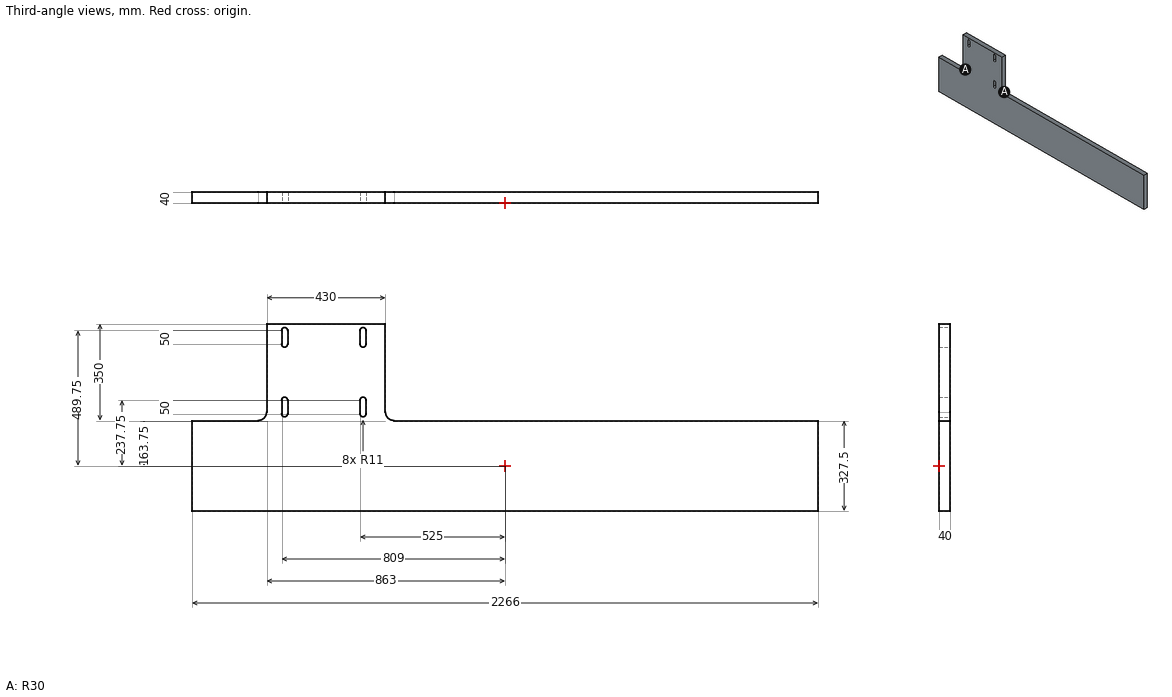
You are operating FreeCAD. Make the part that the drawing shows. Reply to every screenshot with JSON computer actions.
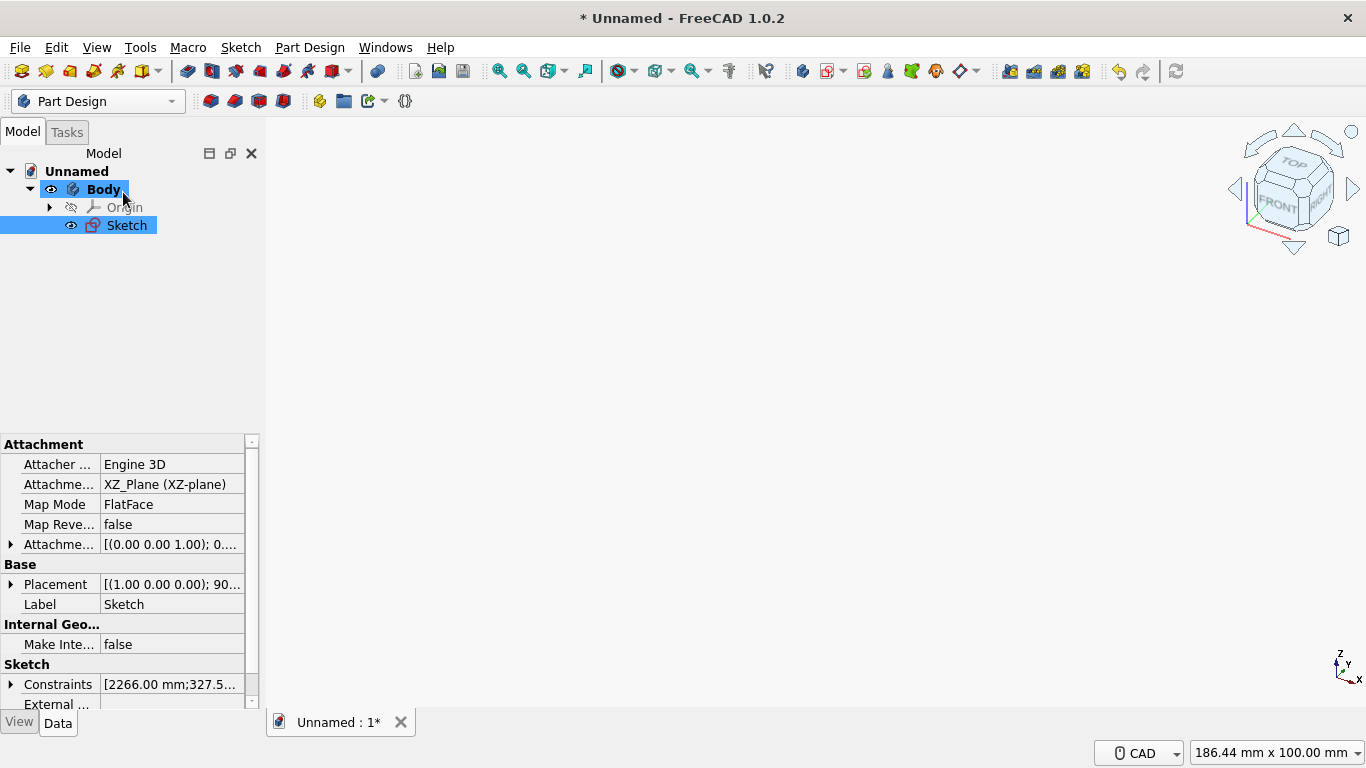
{"action": "left_click", "coordinate": [22, 72]}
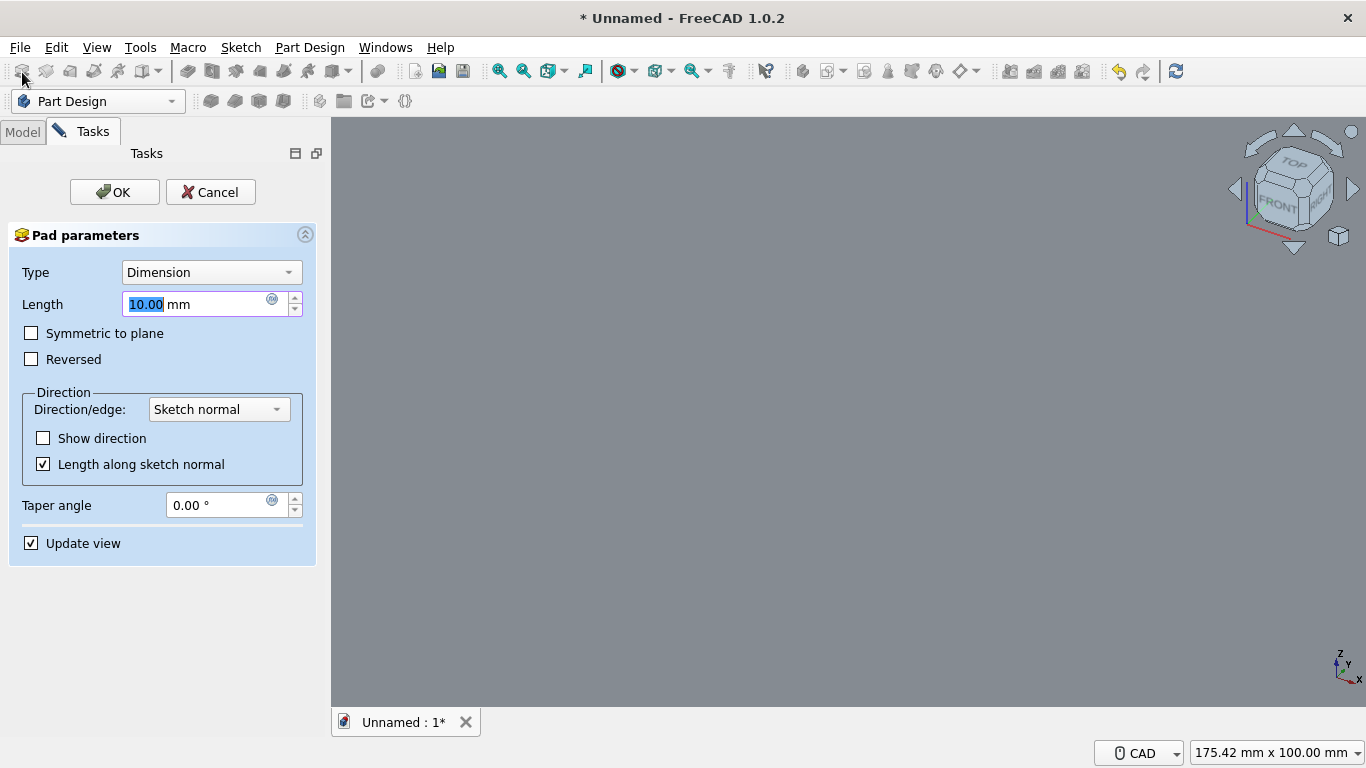
{"action": "type", "text": "40"}
{"action": "key", "text": "Tab"}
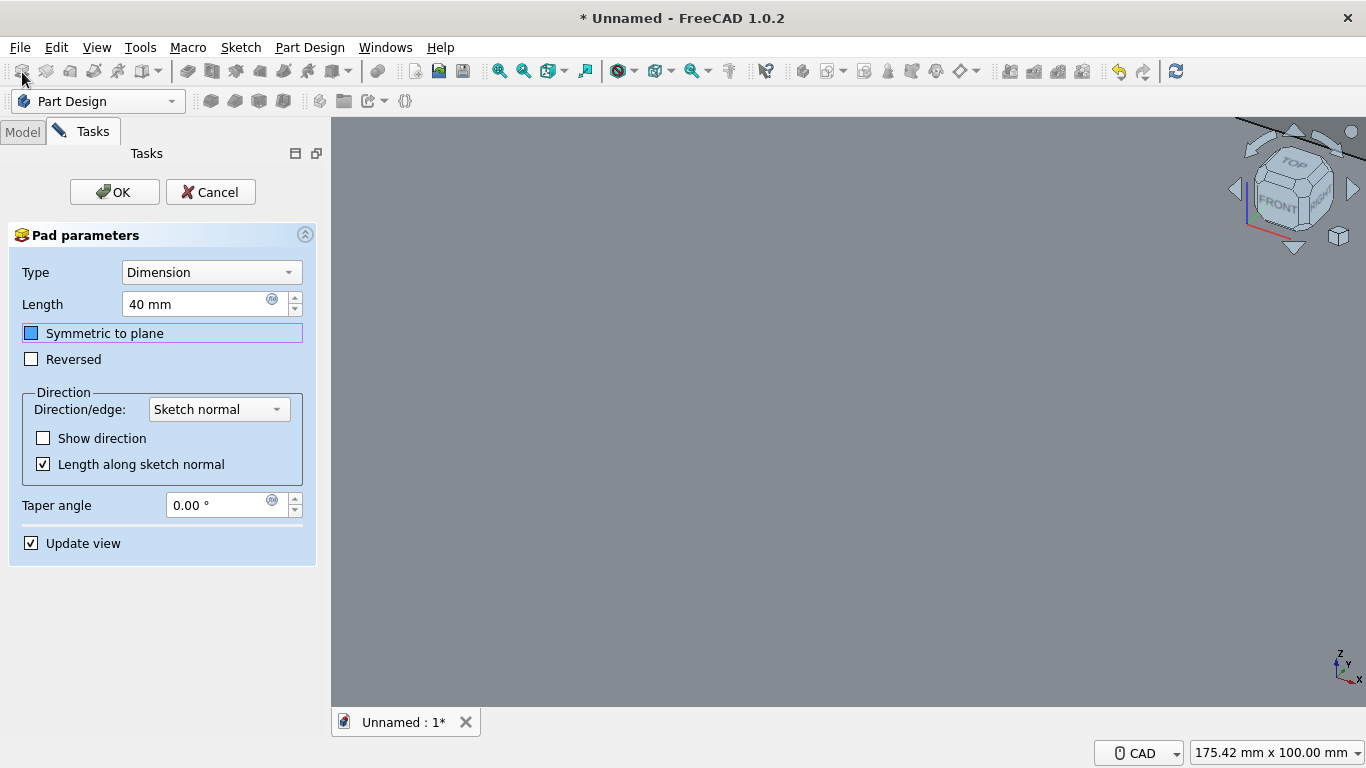
{"action": "left_click", "coordinate": [30, 359]}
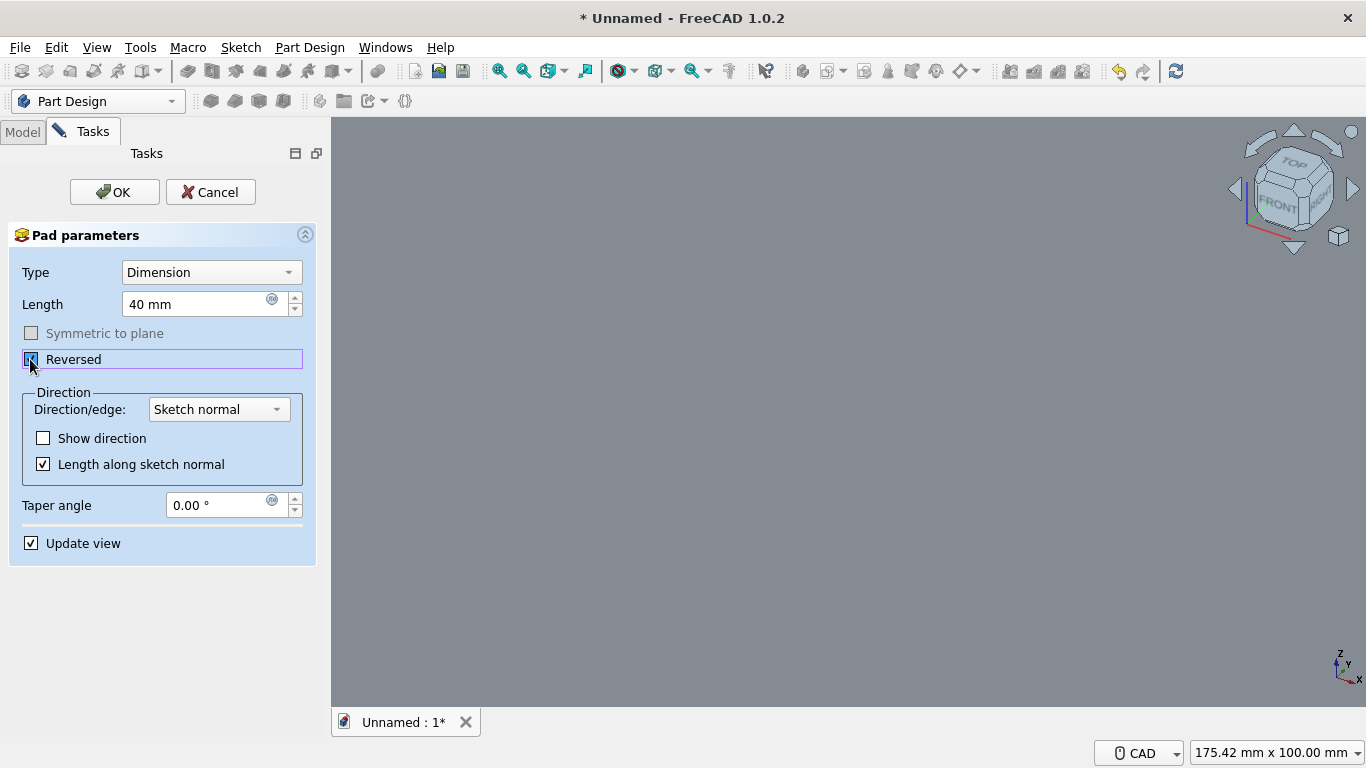
{"action": "left_click", "coordinate": [115, 192]}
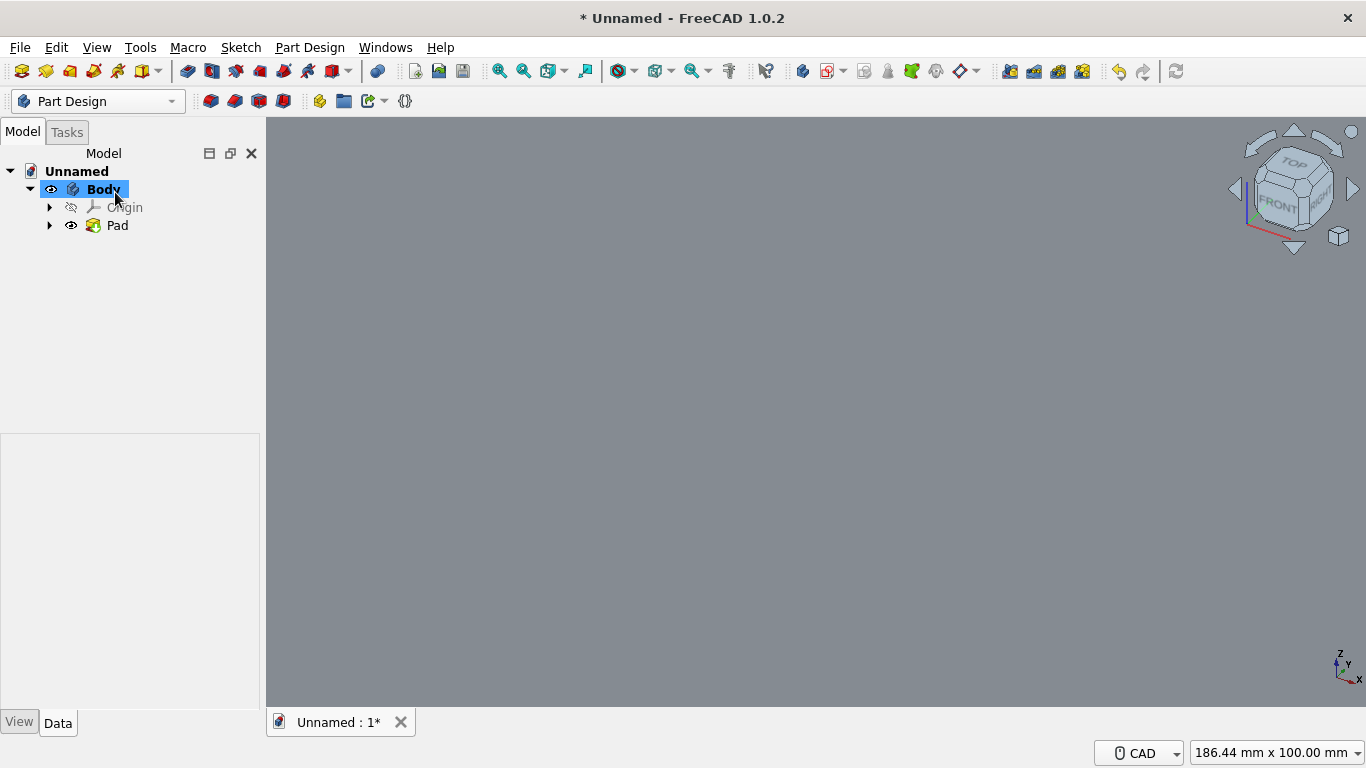
{"action": "key", "text": "v f"}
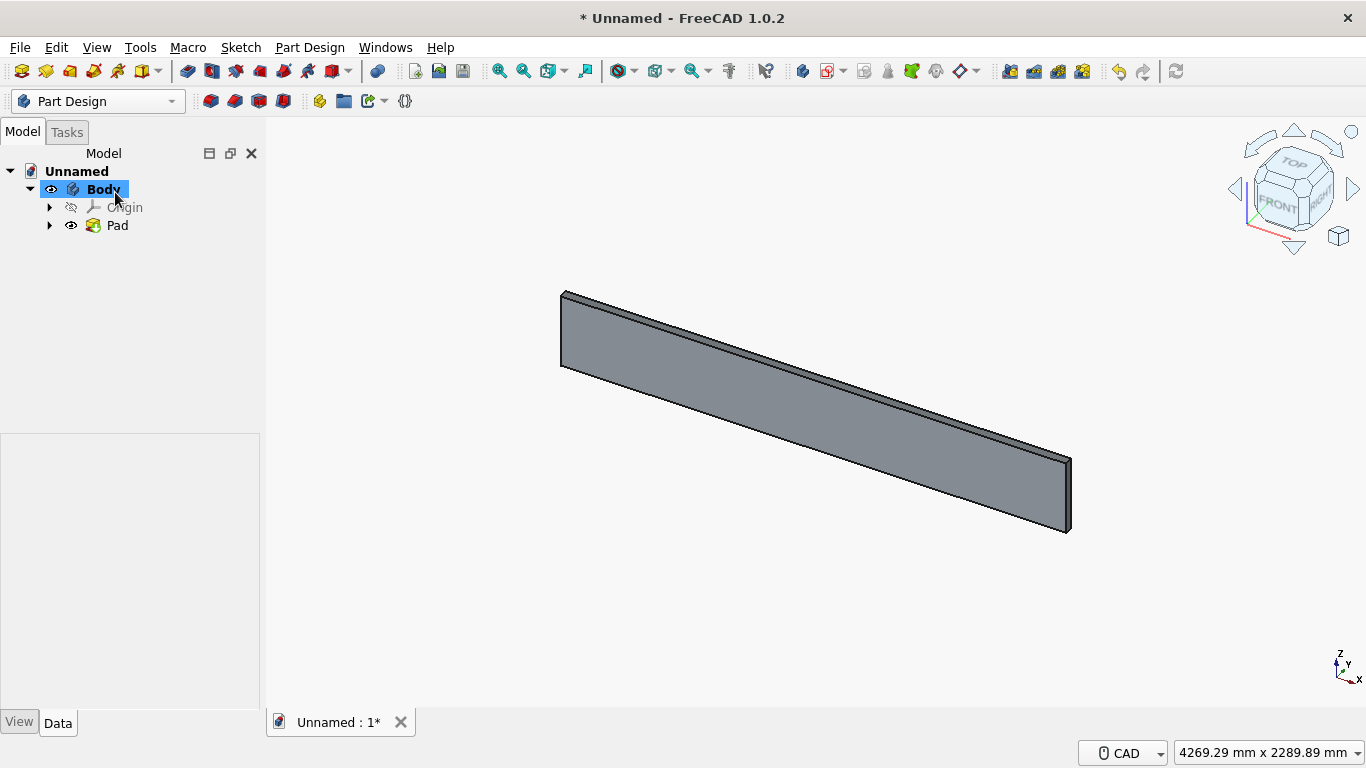
{"action": "key", "text": "4"}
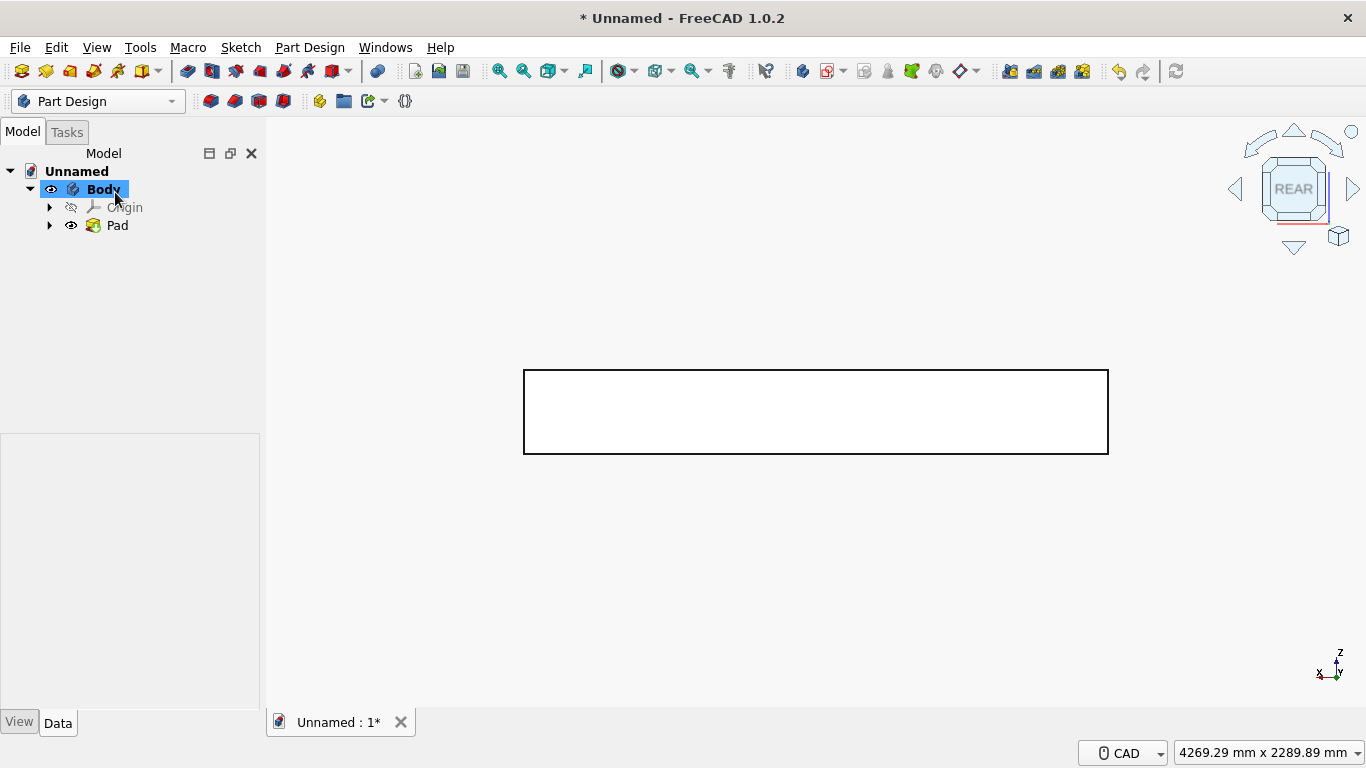
{"action": "left_click", "coordinate": [649, 411]}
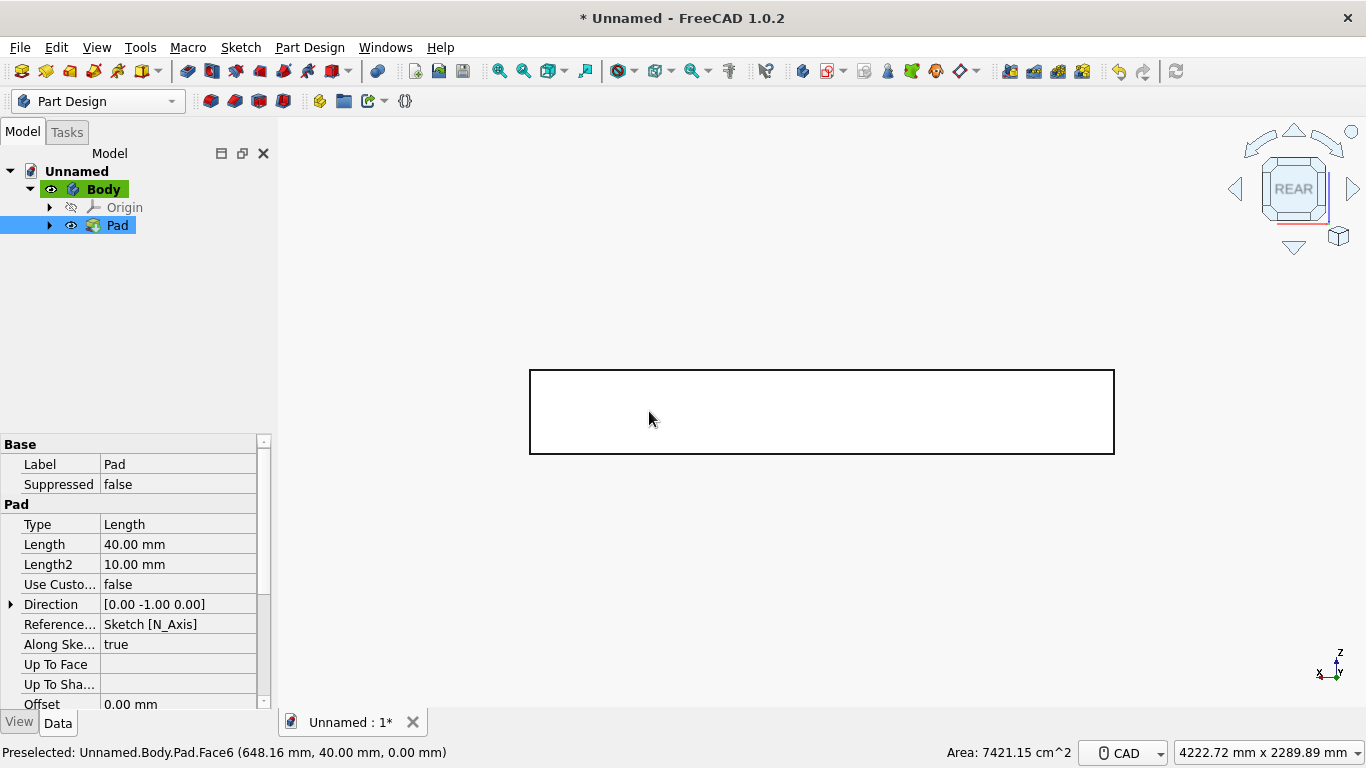
{"action": "left_click", "coordinate": [828, 72]}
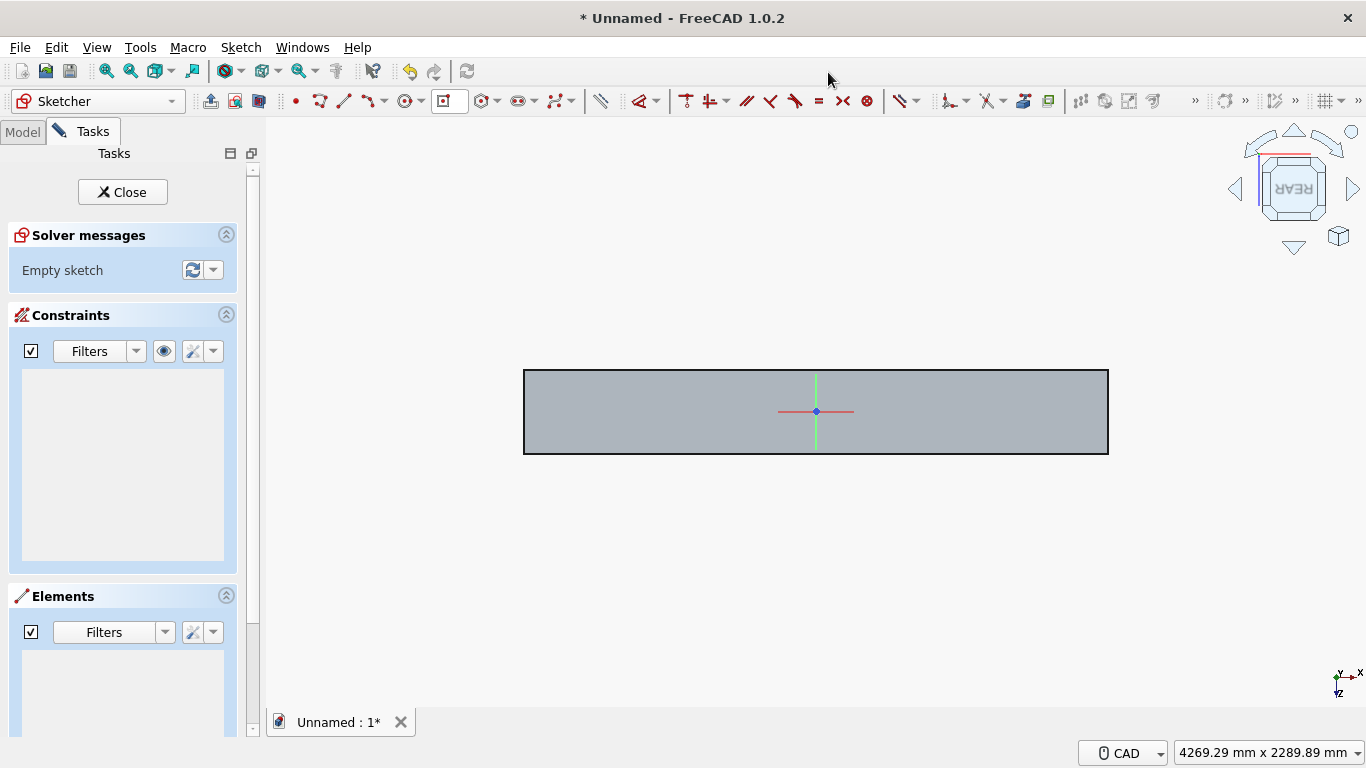
{"action": "scroll", "coordinate": [680, 517], "scroll_direction": "up", "scroll_amount": 5}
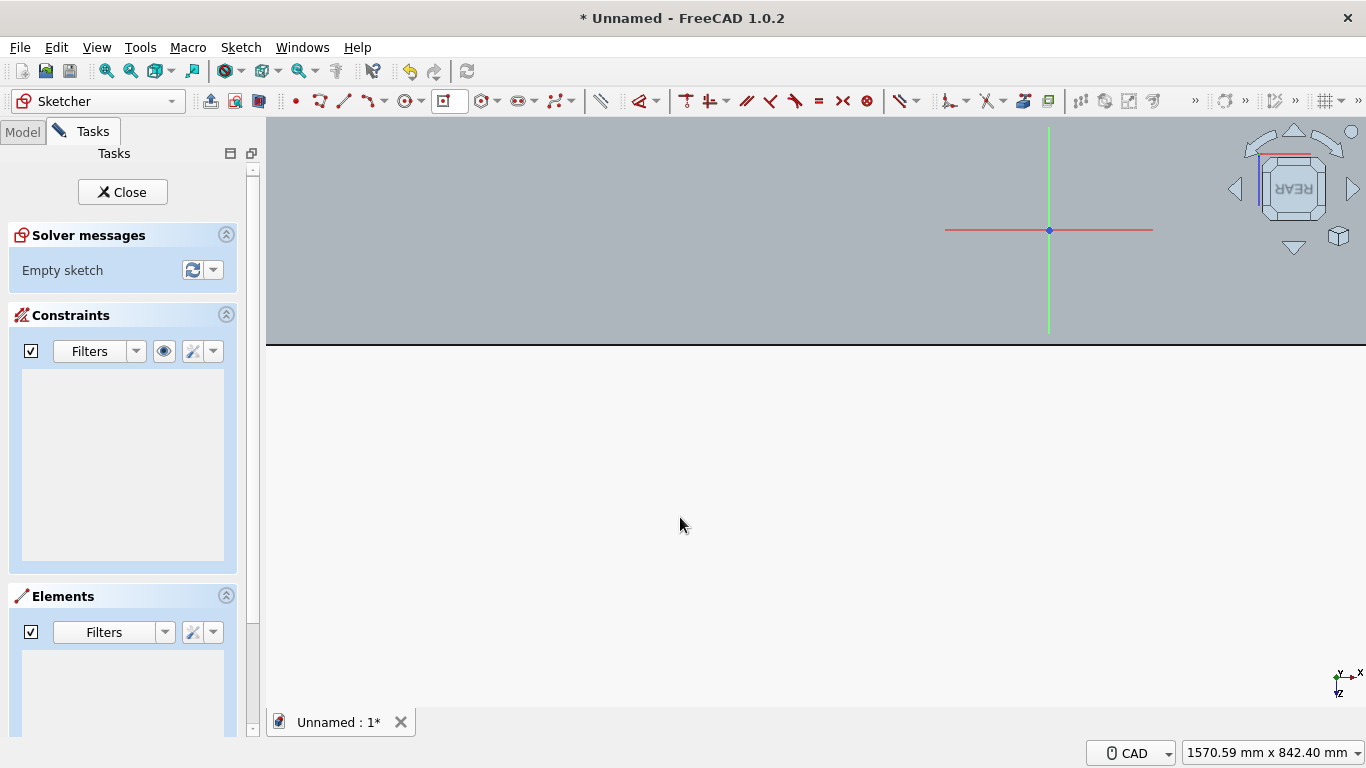
{"action": "key", "text": "g r"}